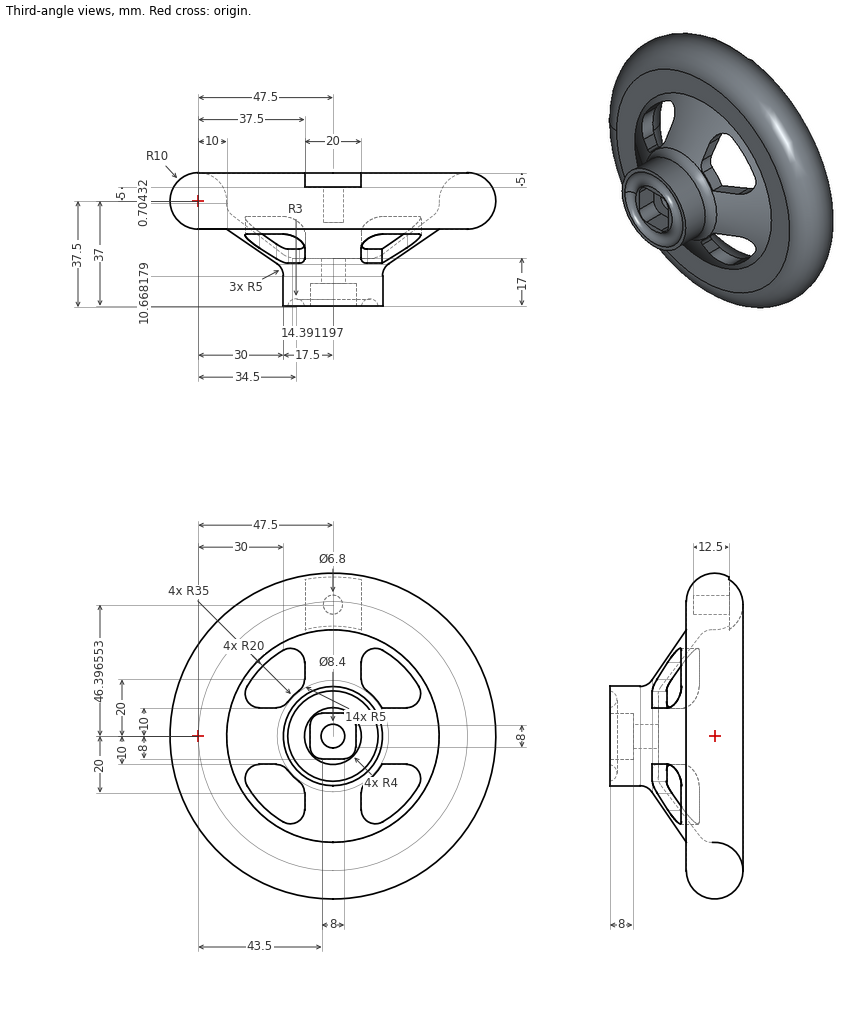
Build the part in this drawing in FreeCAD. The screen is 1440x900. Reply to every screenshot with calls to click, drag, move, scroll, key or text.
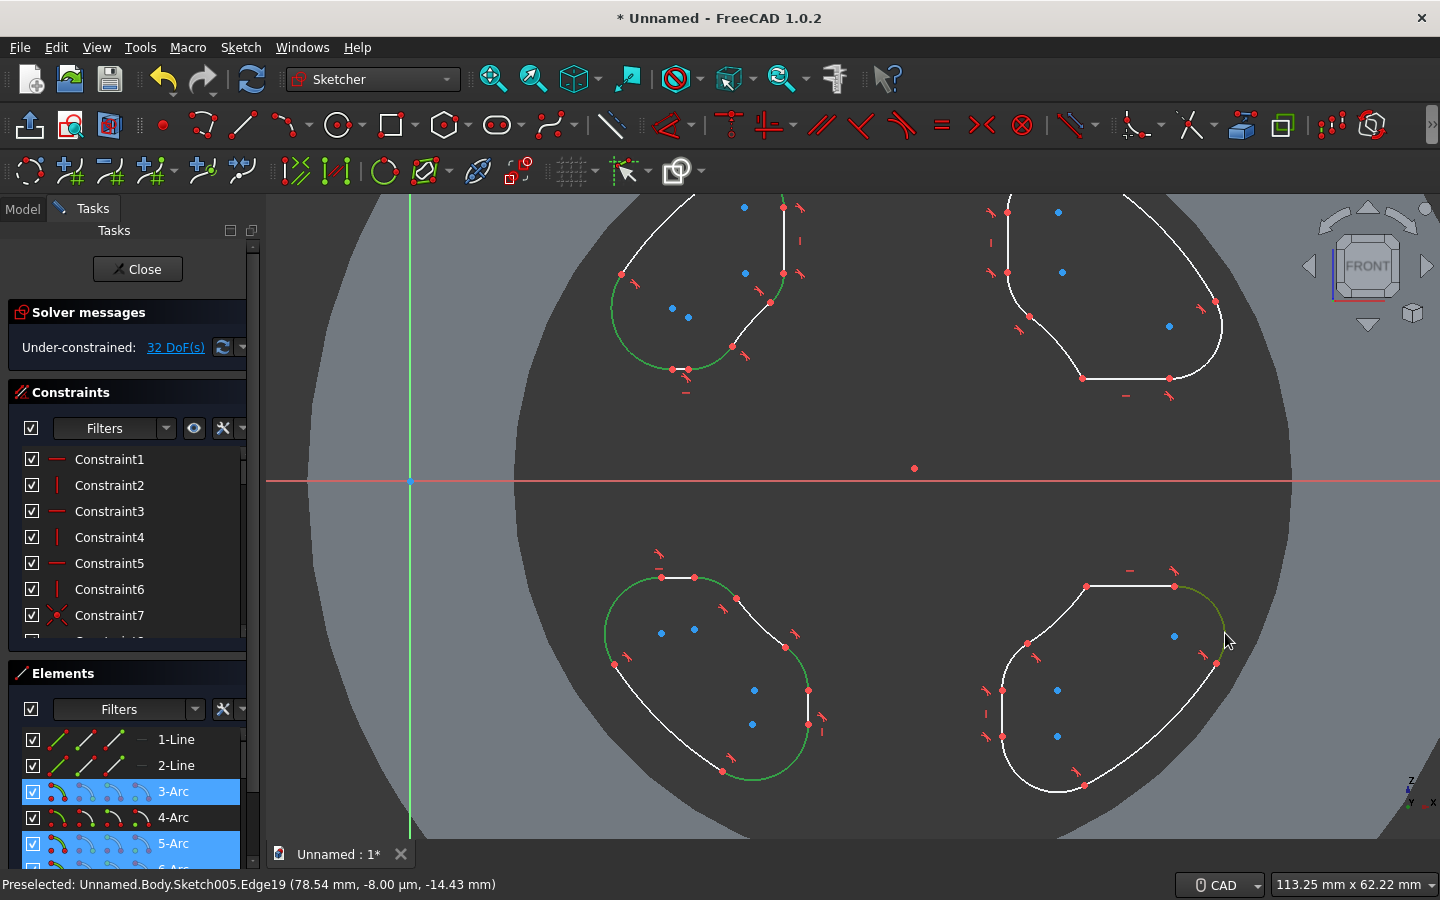
click(1012, 769)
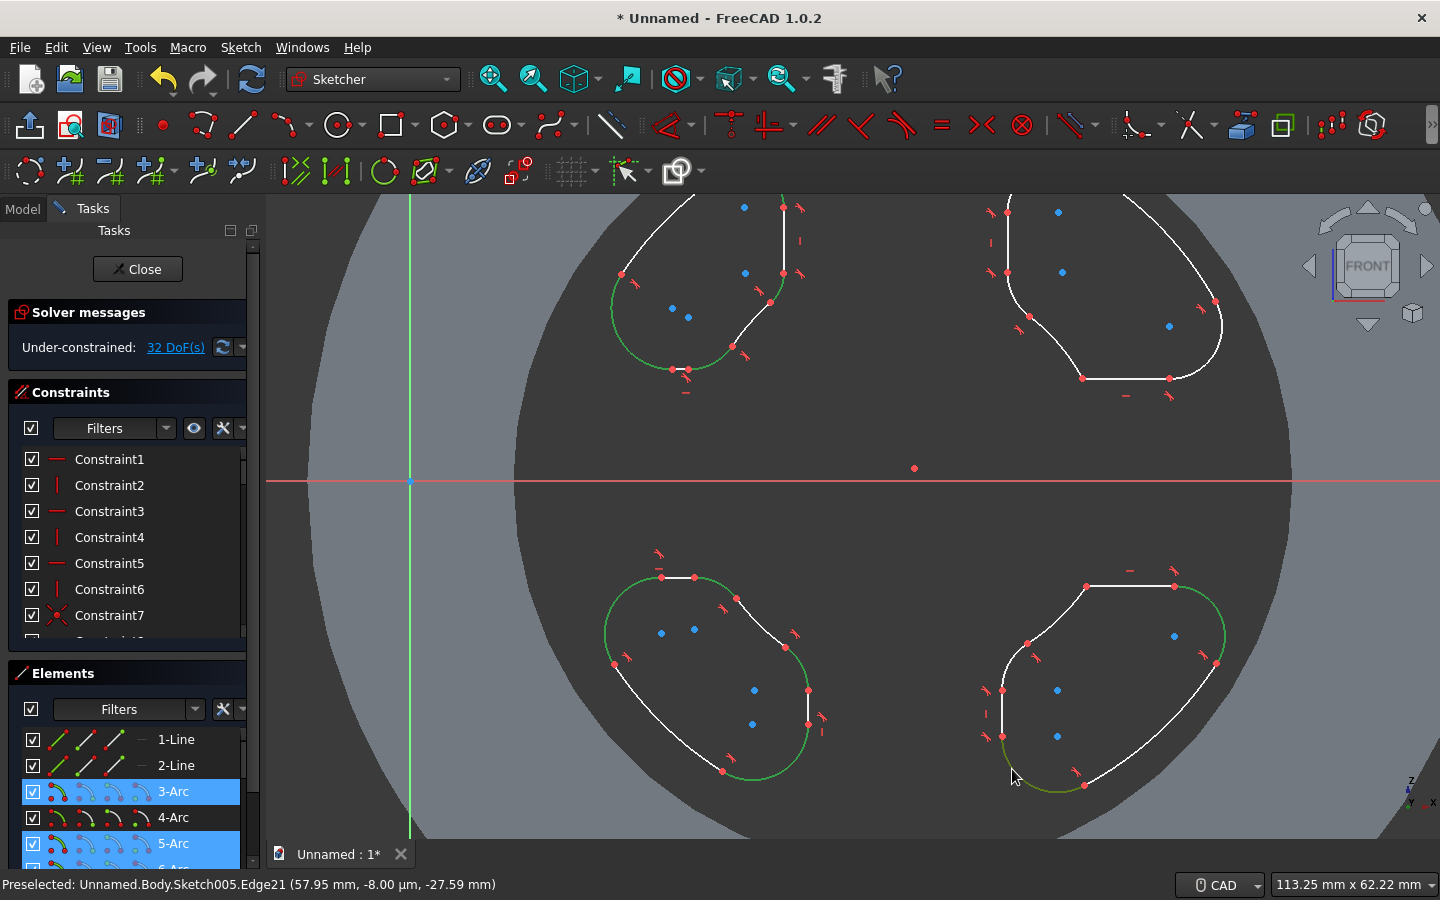
click(1015, 655)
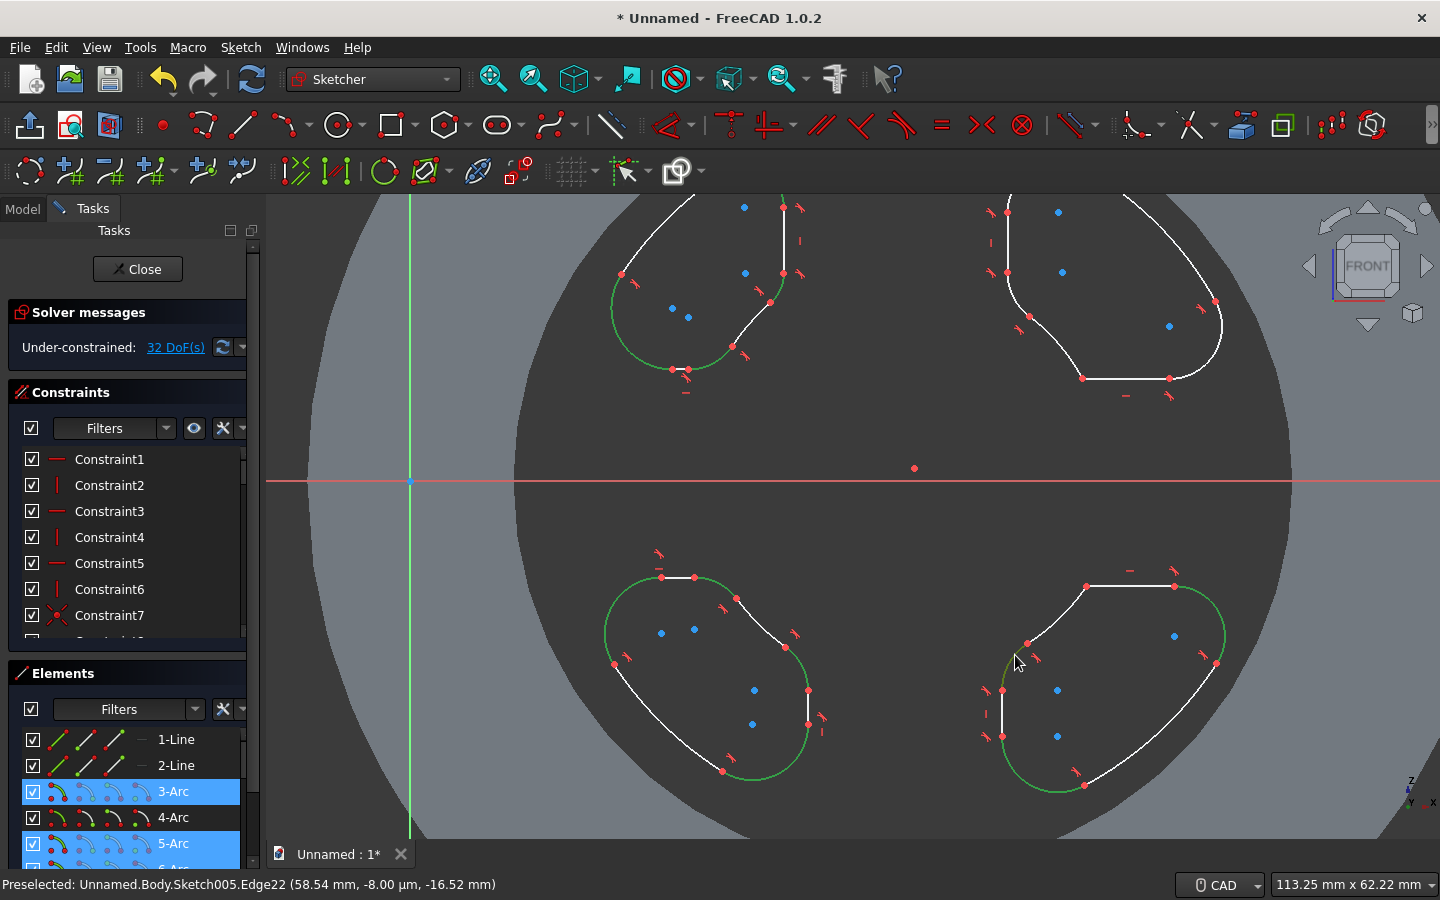
click(1010, 287)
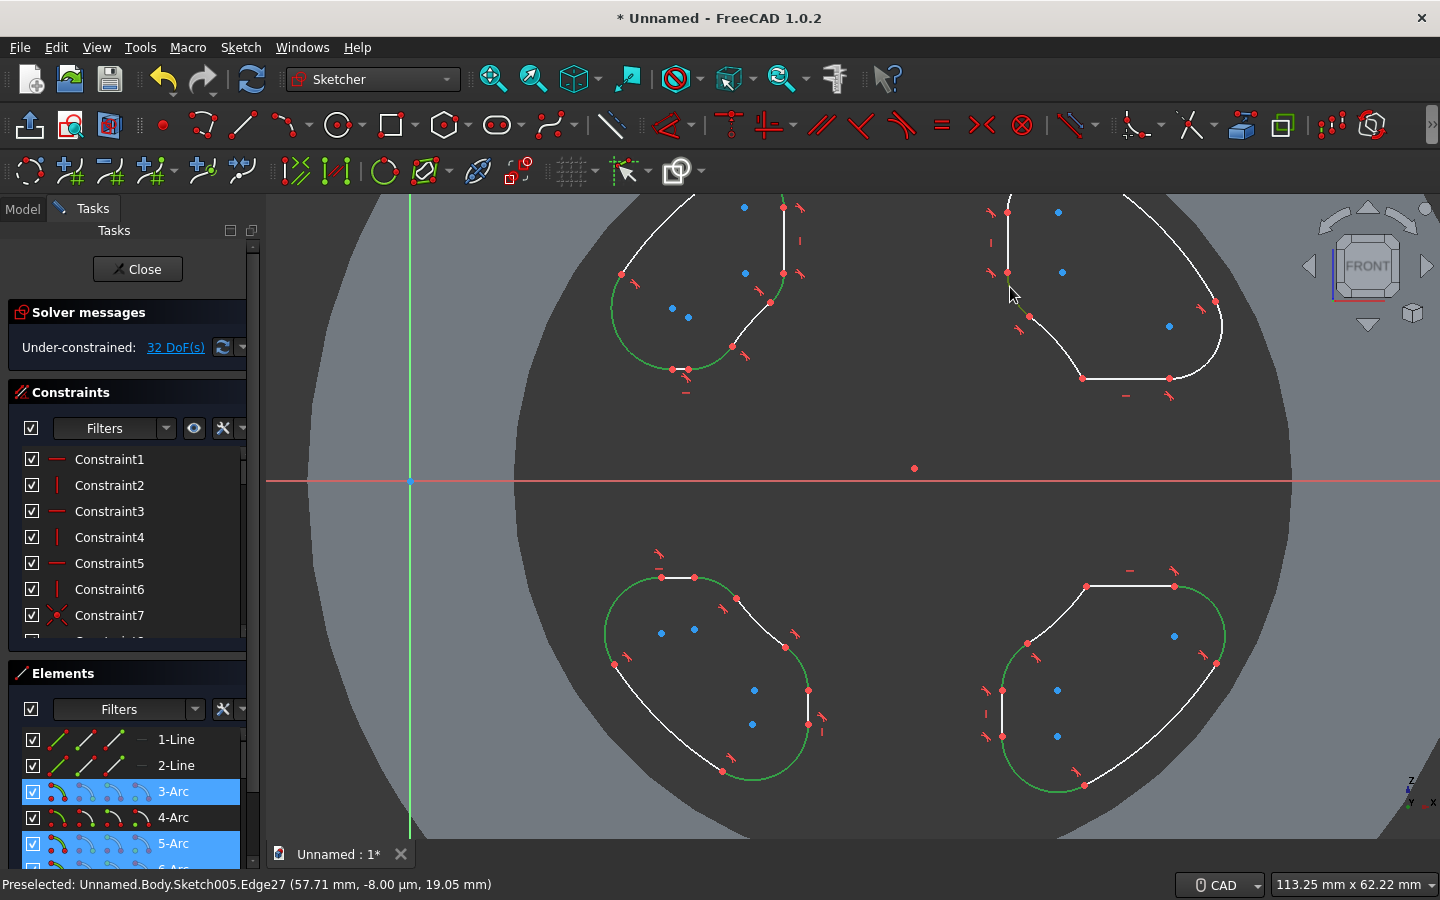
scroll(725, 589, down, 2)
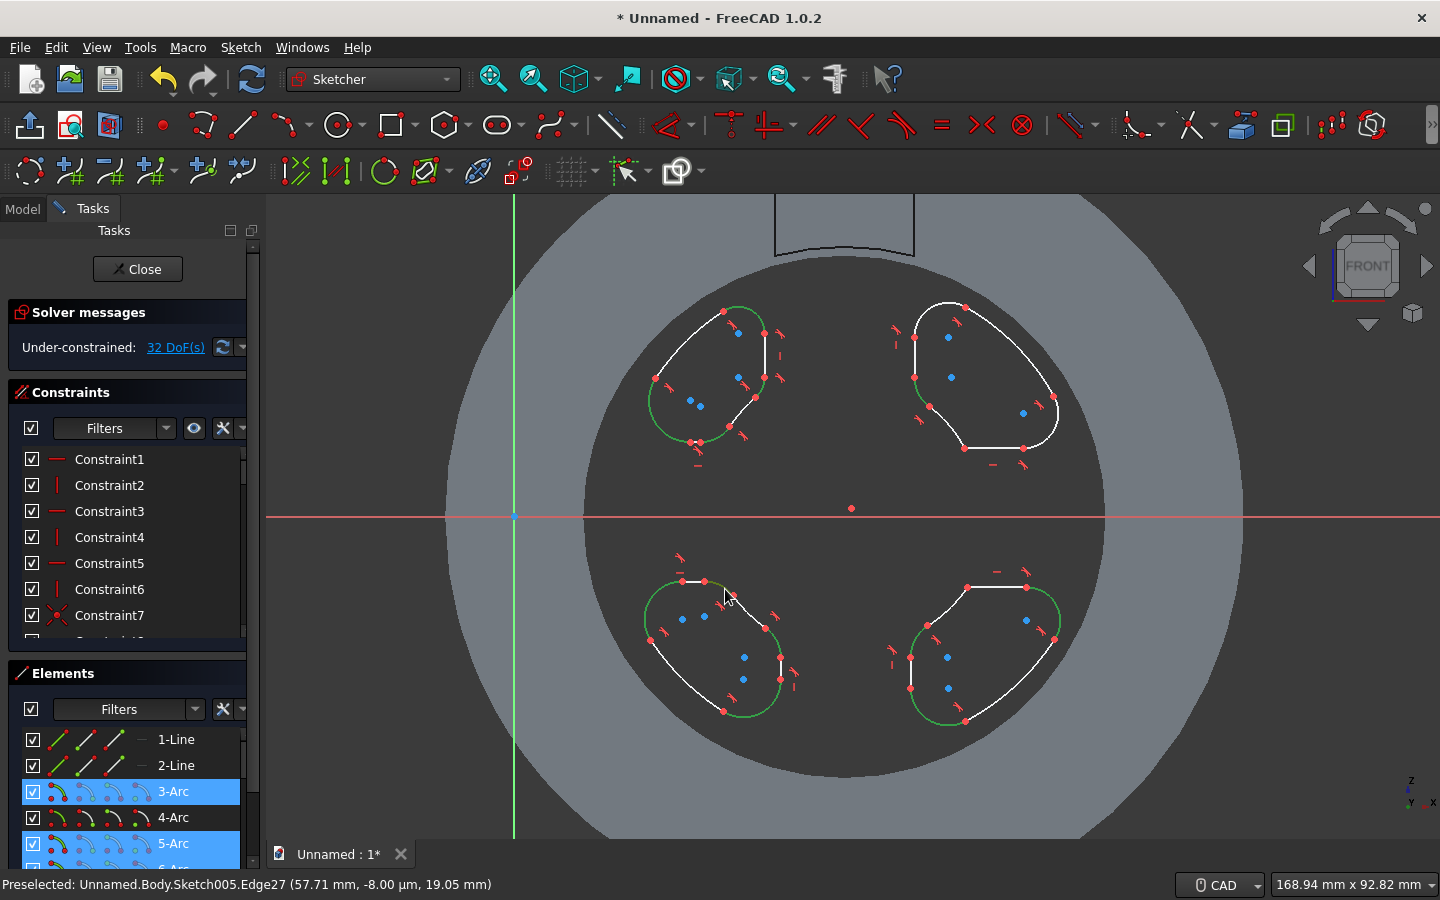
click(945, 303)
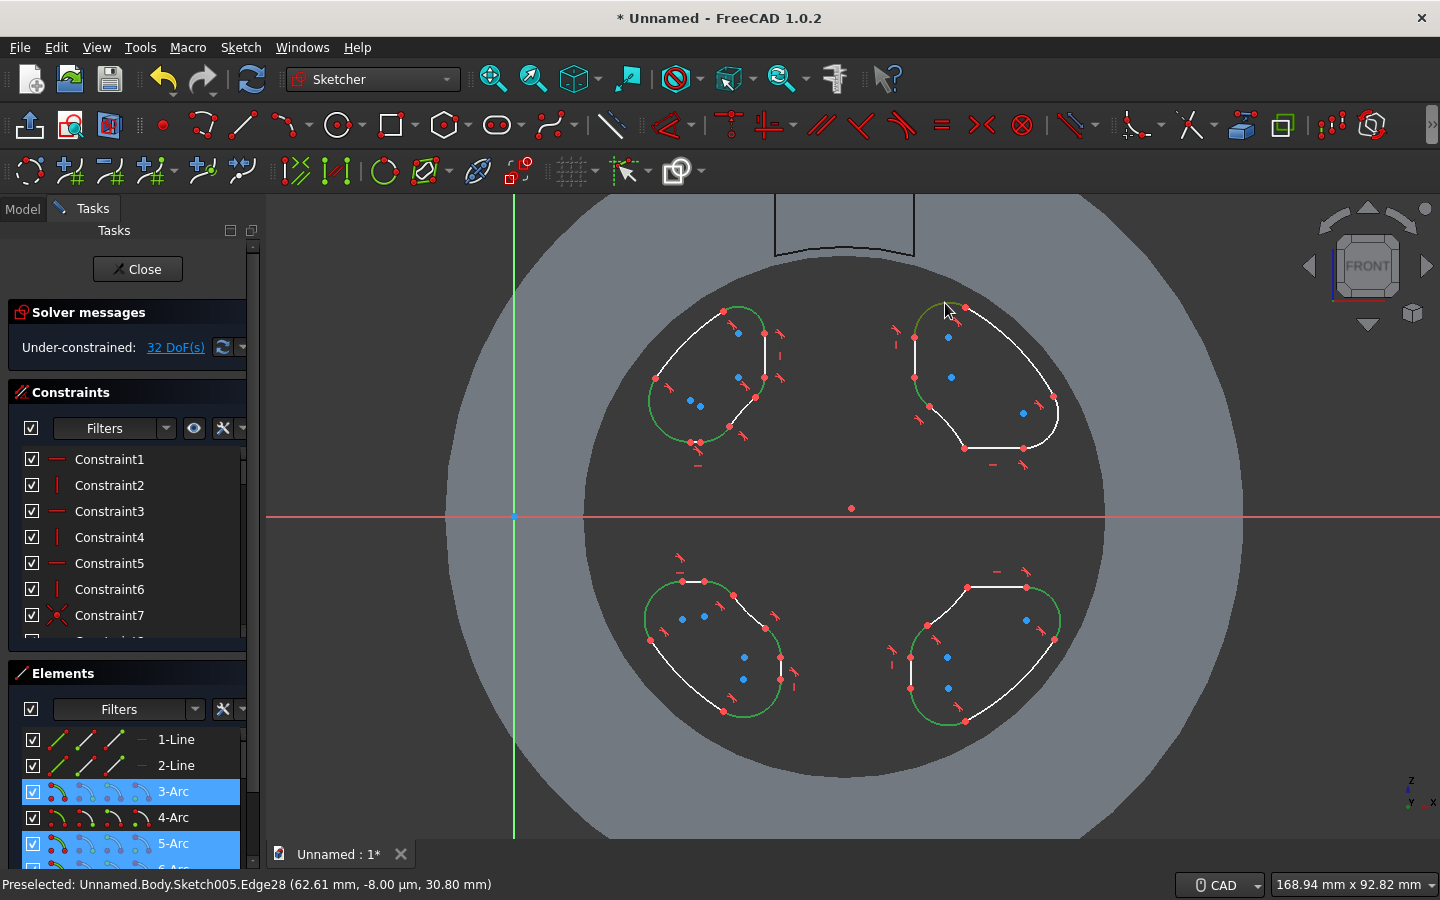
click(1044, 442)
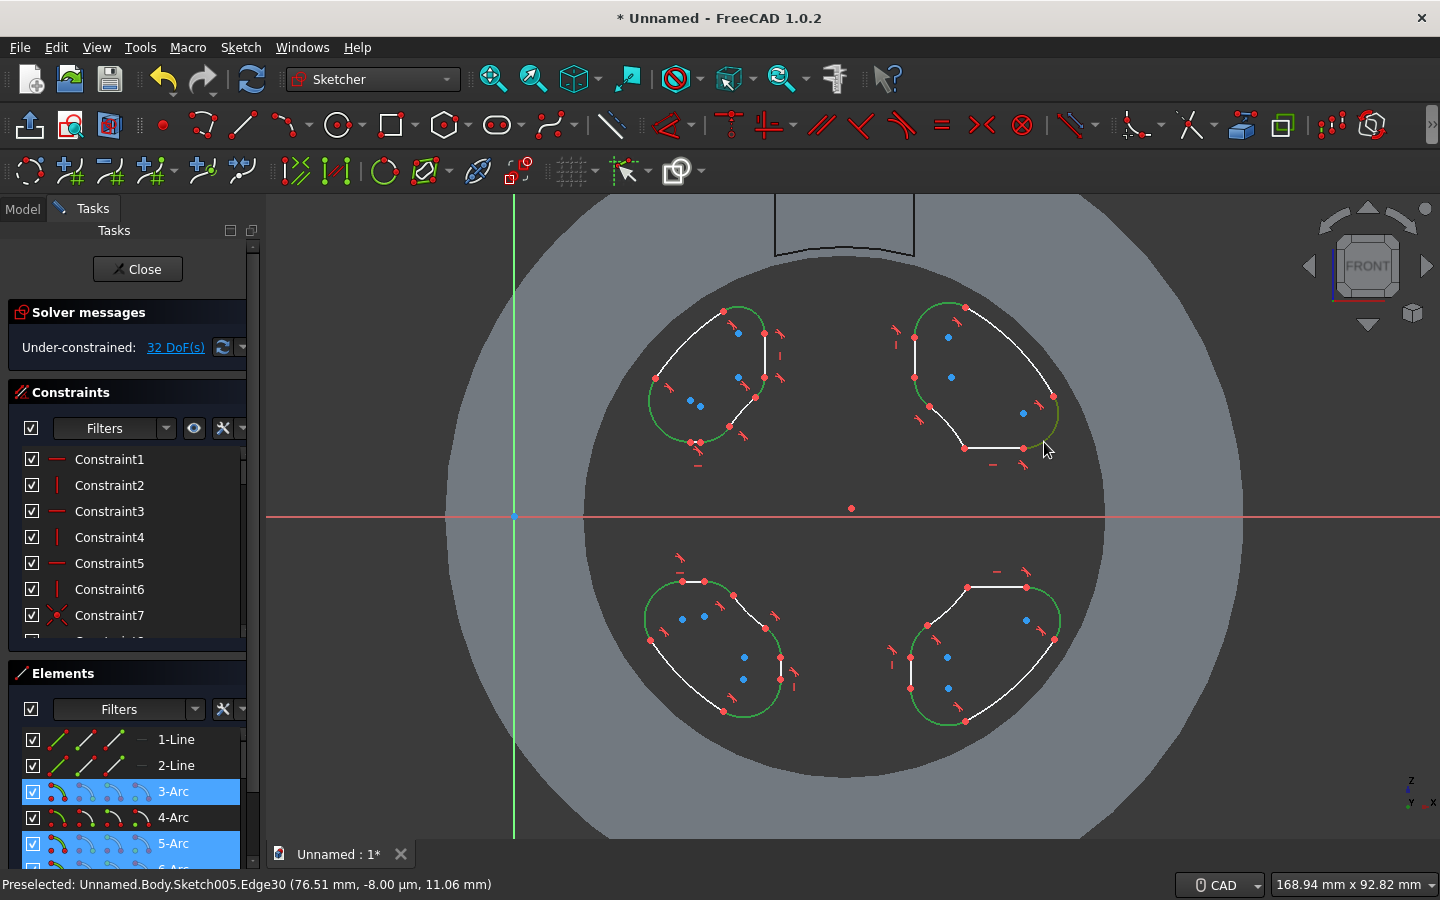
click(942, 126)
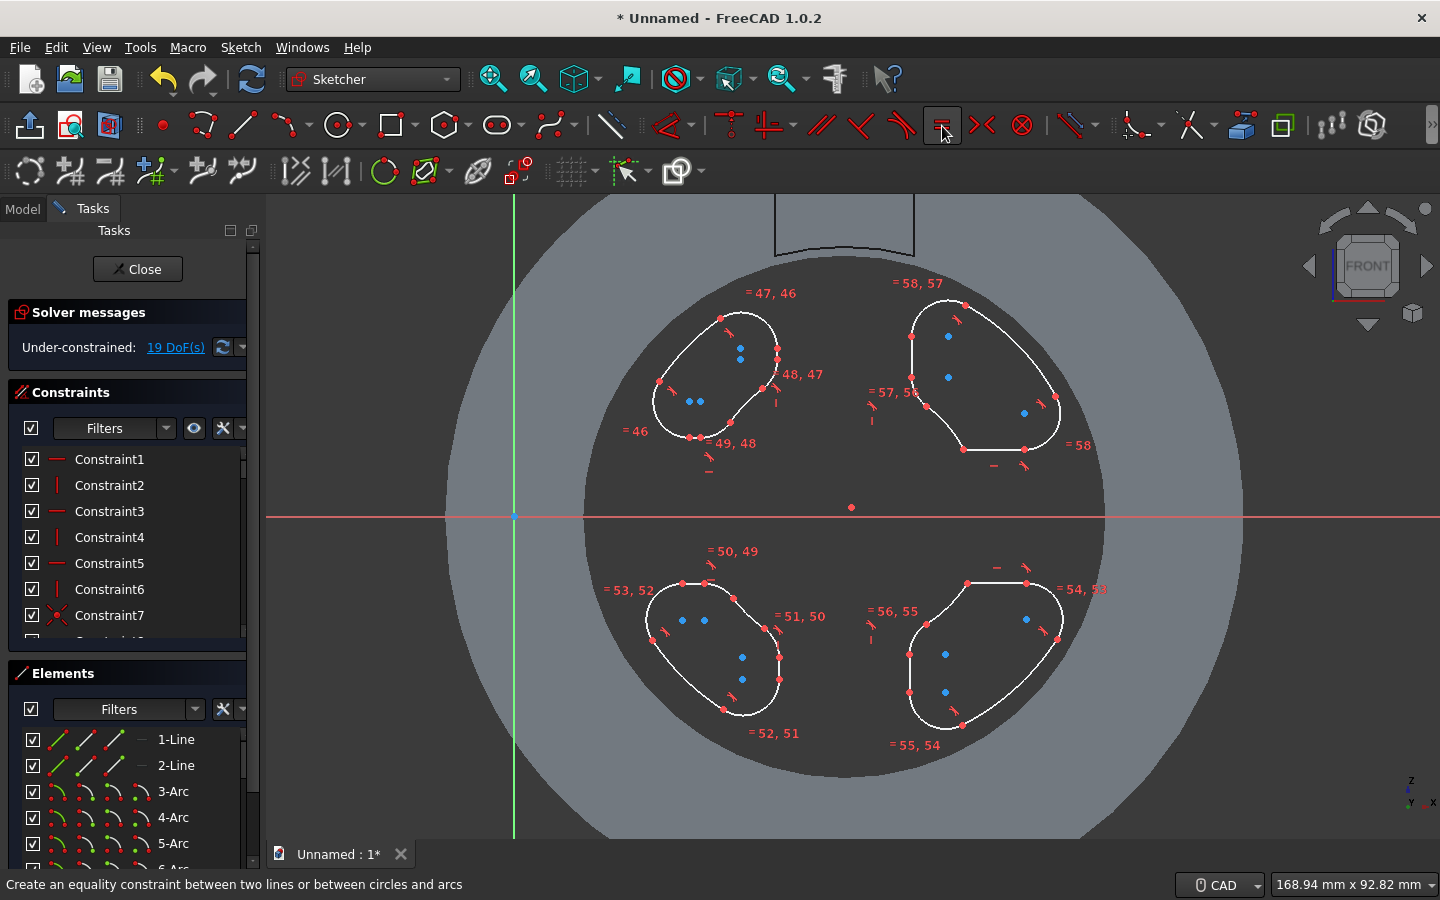
click(752, 398)